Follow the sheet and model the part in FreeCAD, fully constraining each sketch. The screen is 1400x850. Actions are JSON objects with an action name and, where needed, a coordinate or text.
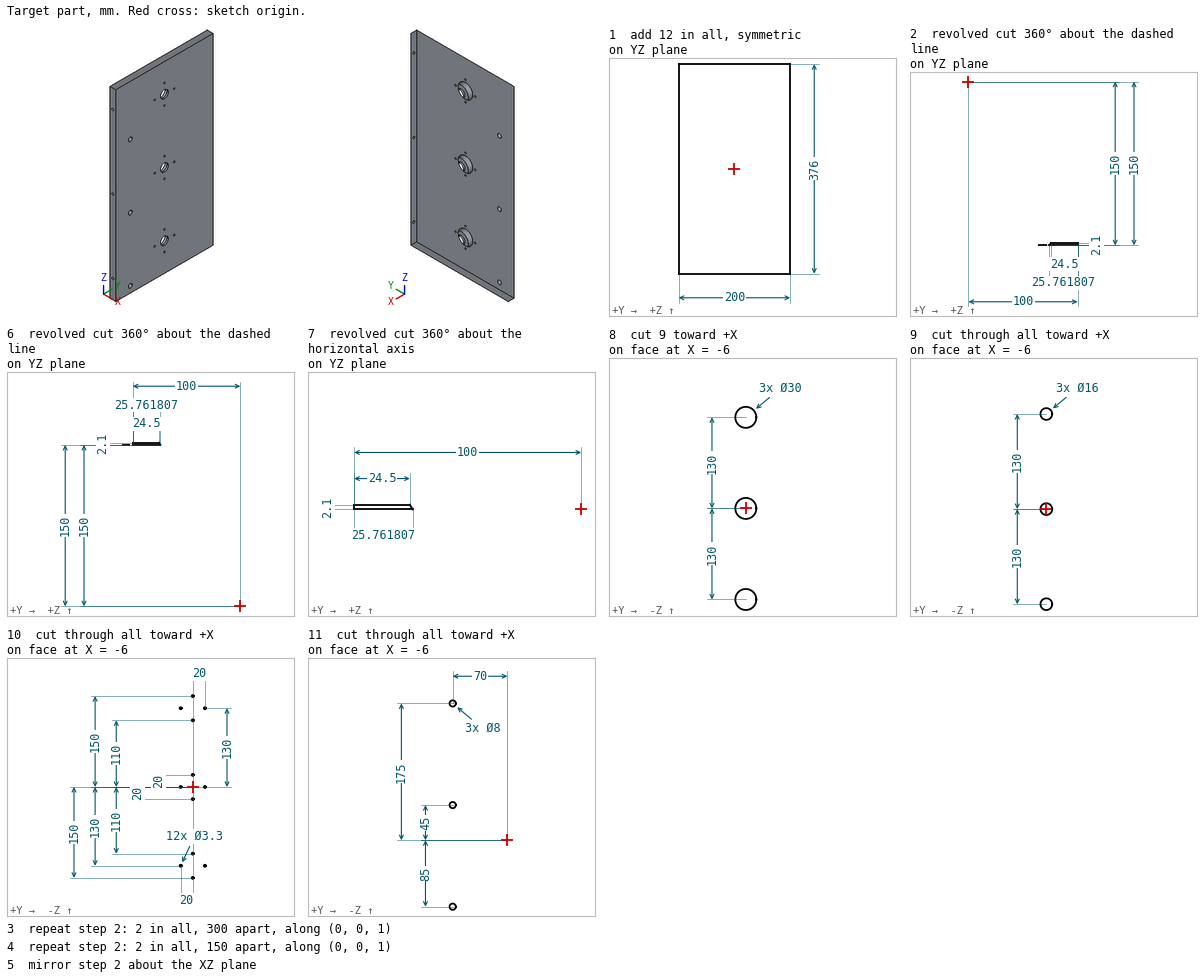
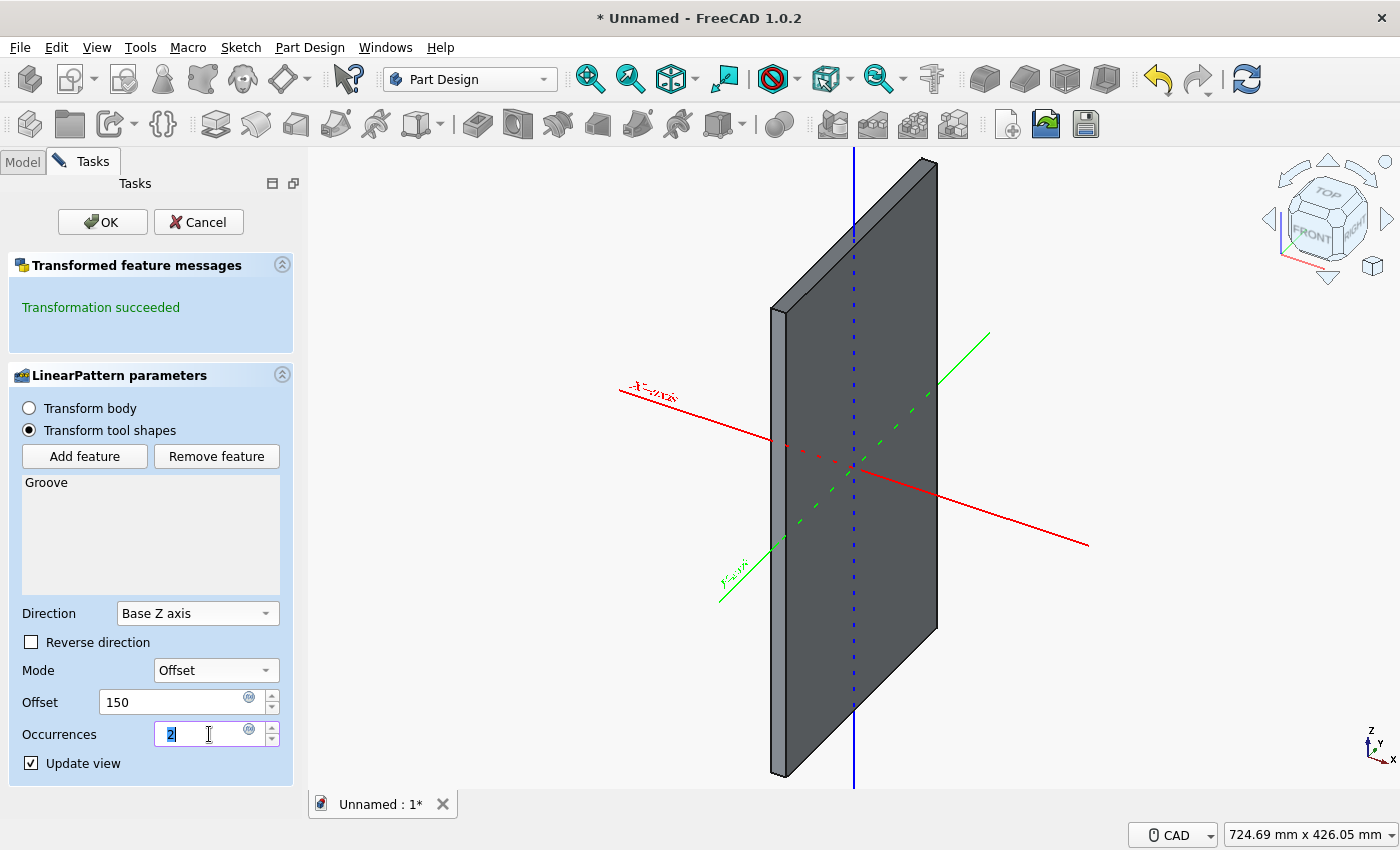
{"action": "type", "text": "2"}
{"action": "key", "text": "Tab"}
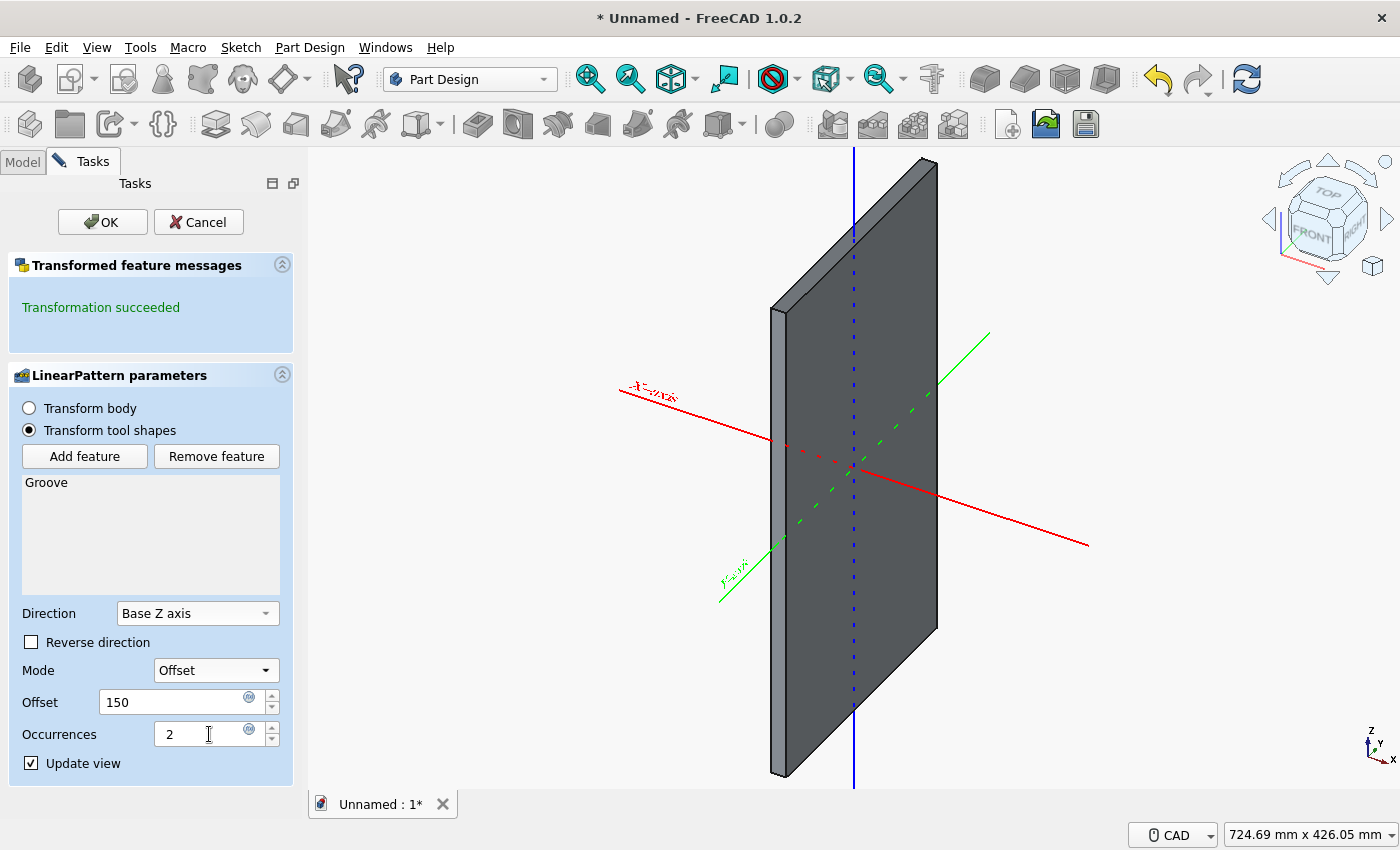
{"action": "left_click", "coordinate": [103, 222]}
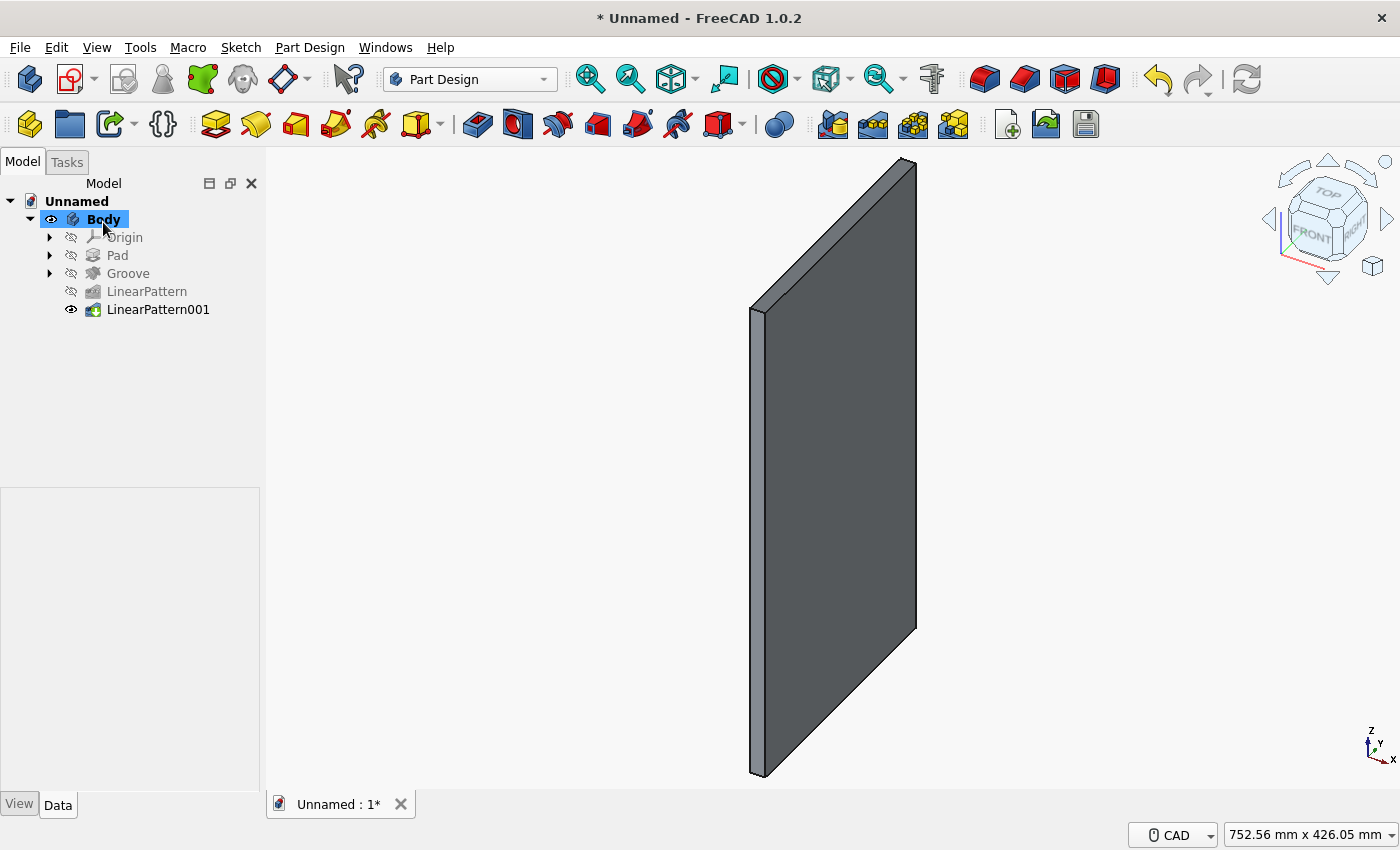
{"action": "left_click", "coordinate": [116, 273]}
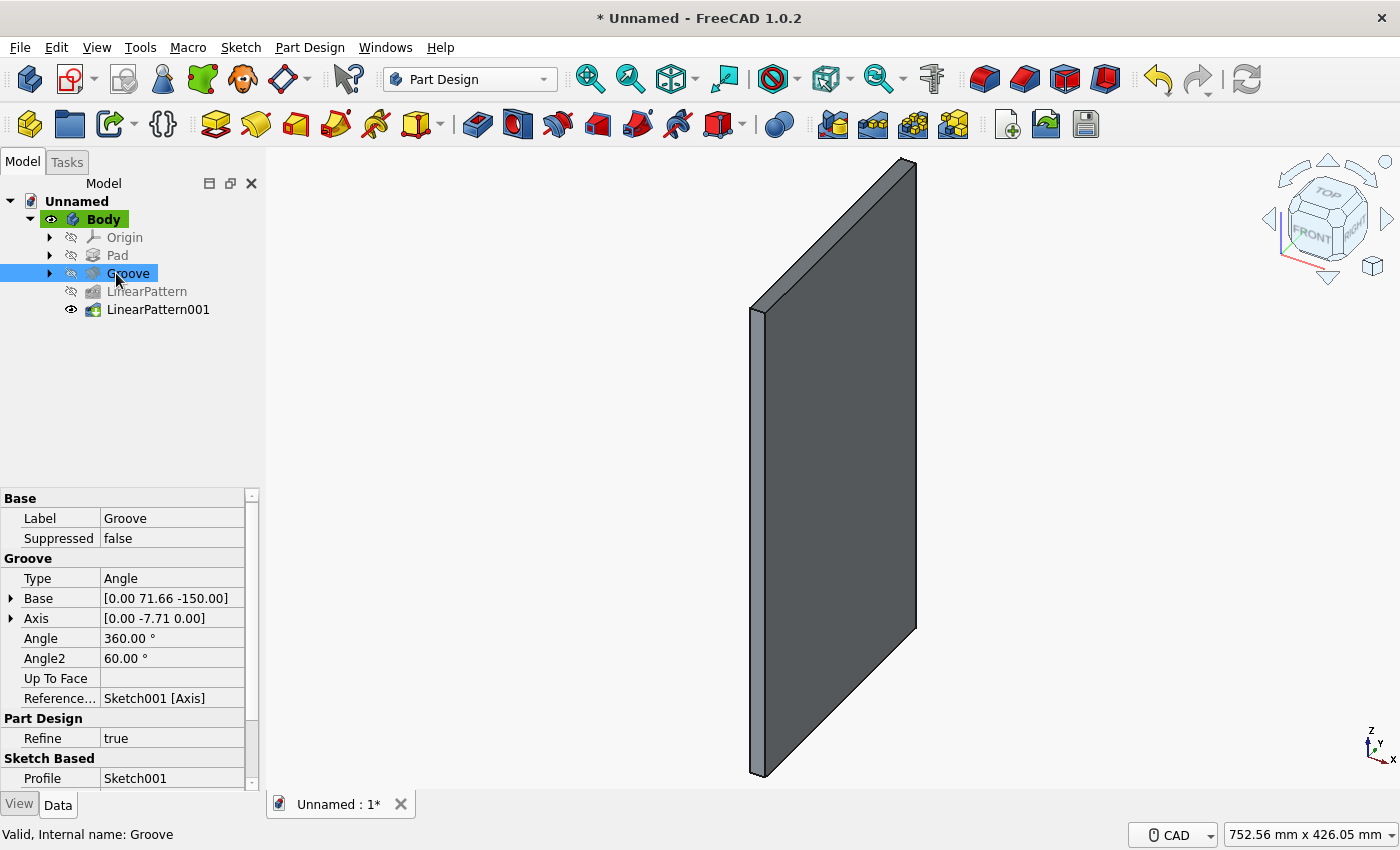
{"action": "left_click", "coordinate": [834, 124]}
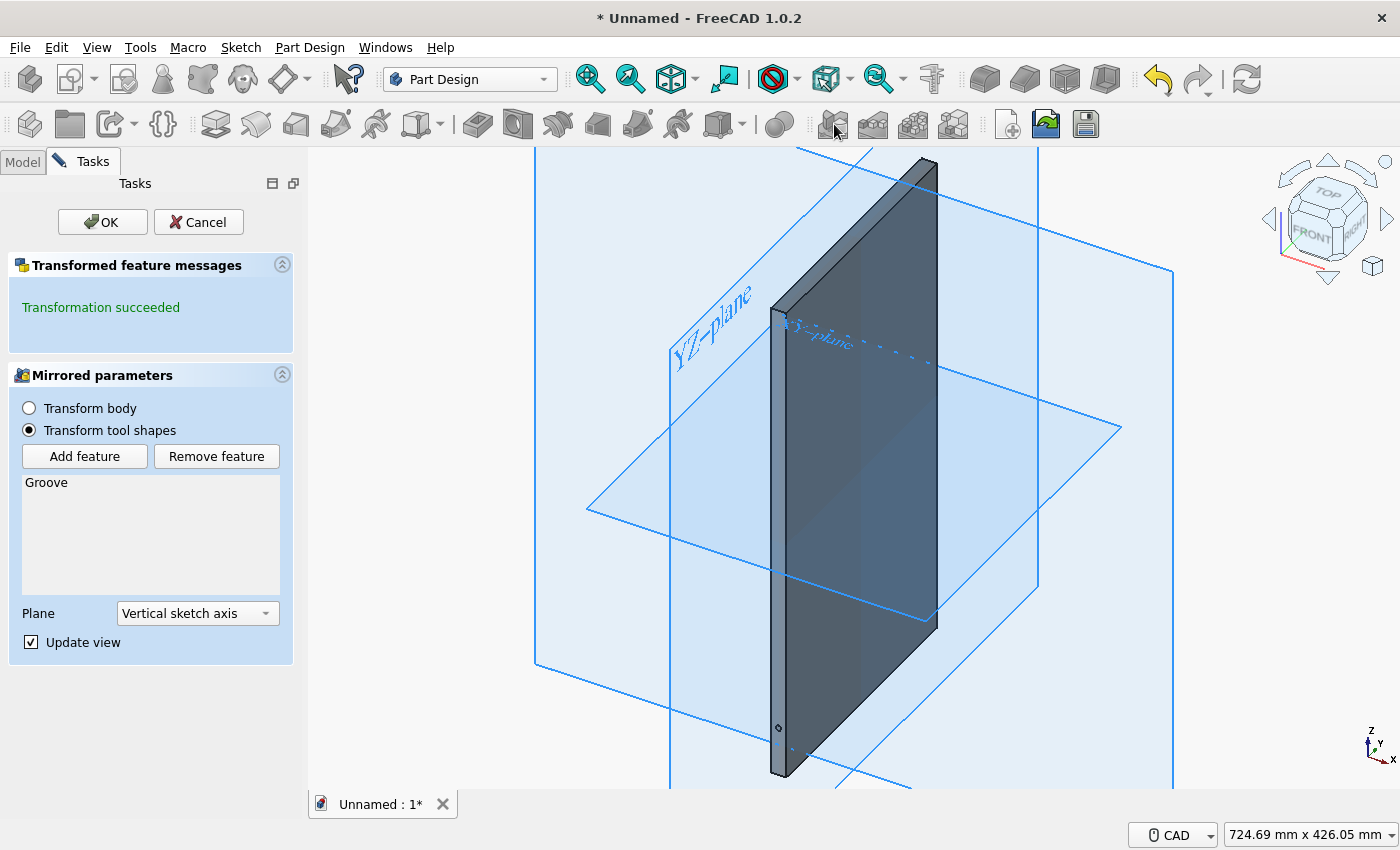
{"action": "left_click", "coordinate": [198, 614]}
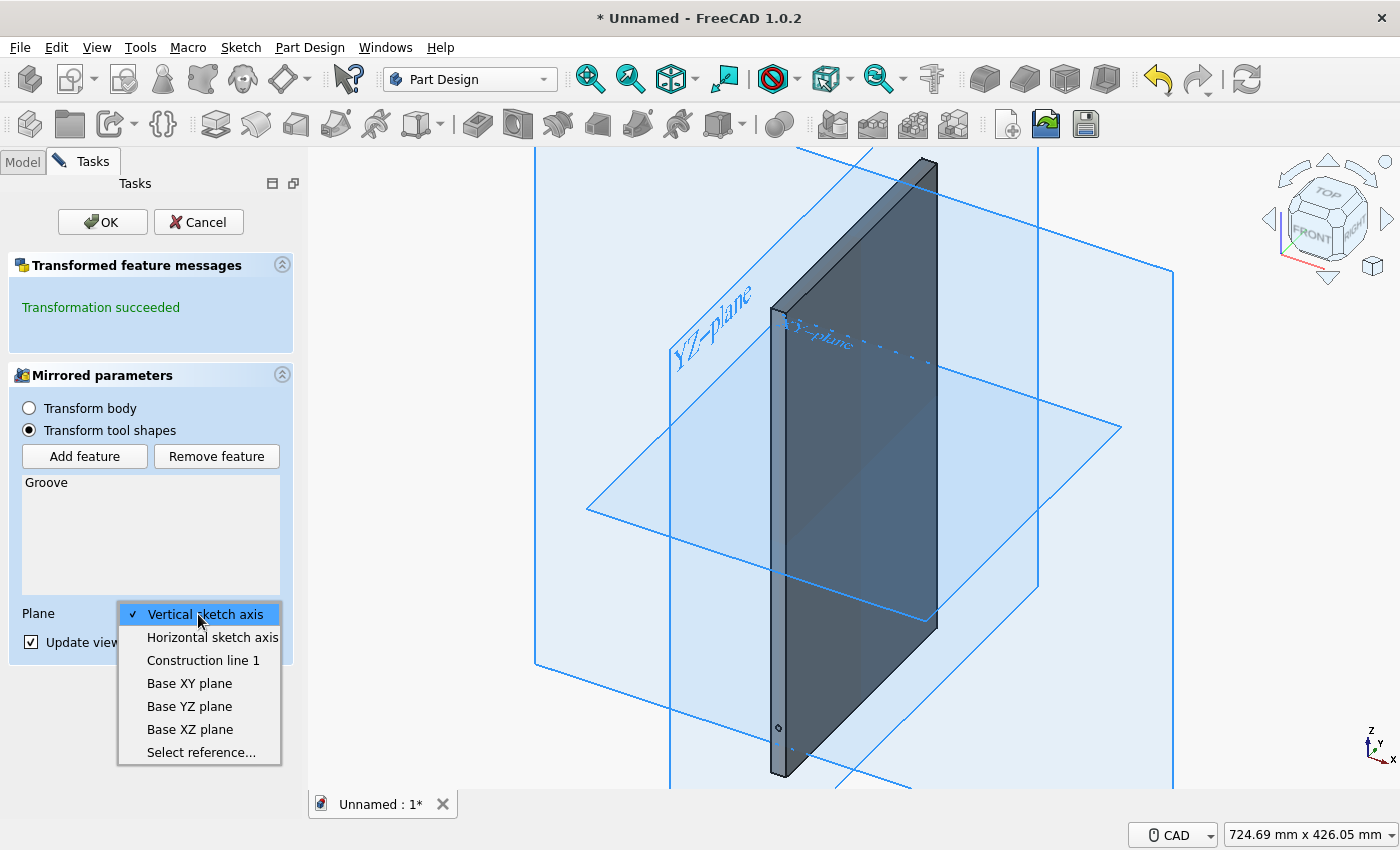
{"action": "left_click", "coordinate": [198, 730]}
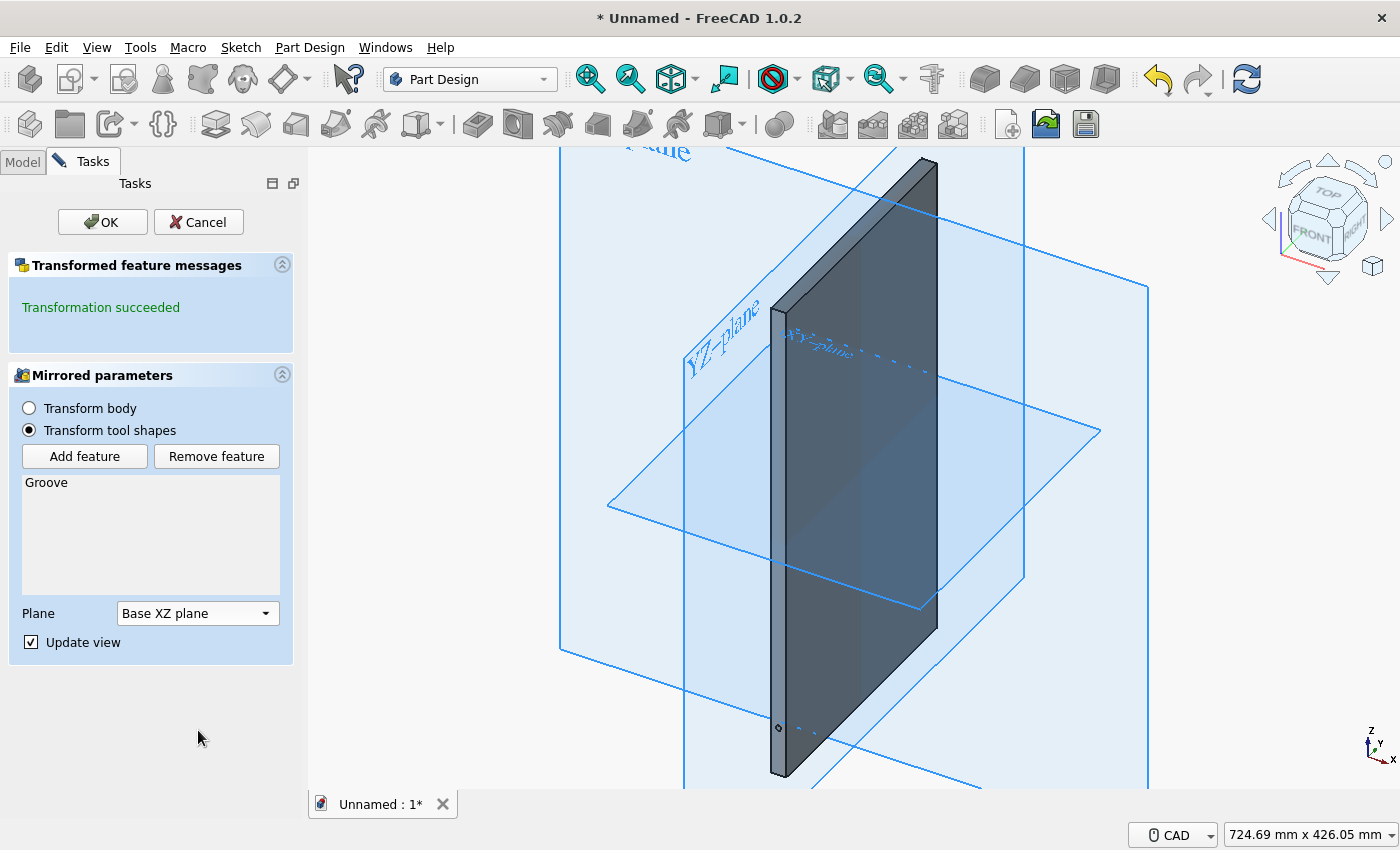
{"action": "left_click", "coordinate": [103, 222]}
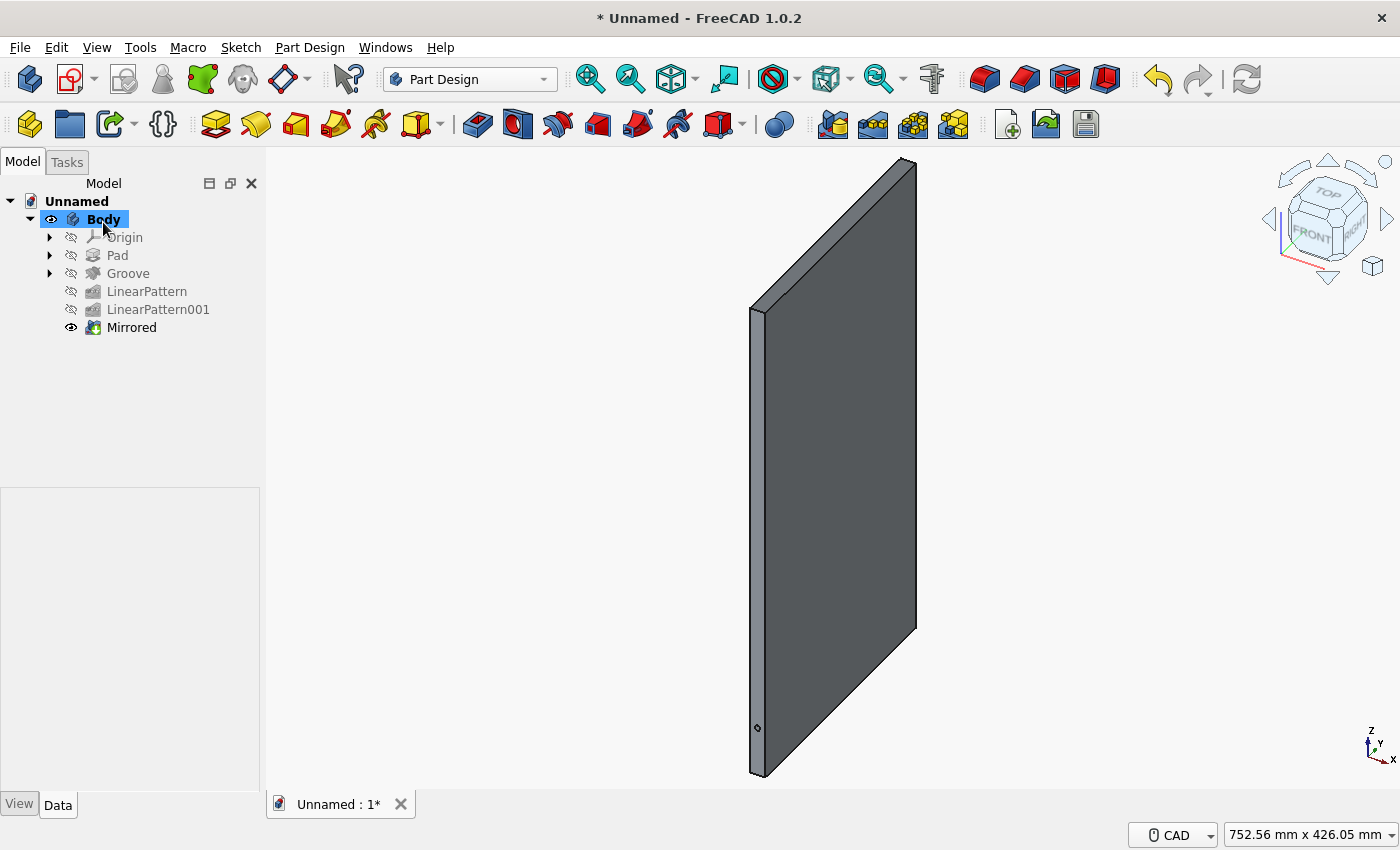
{"action": "left_click", "coordinate": [70, 80]}